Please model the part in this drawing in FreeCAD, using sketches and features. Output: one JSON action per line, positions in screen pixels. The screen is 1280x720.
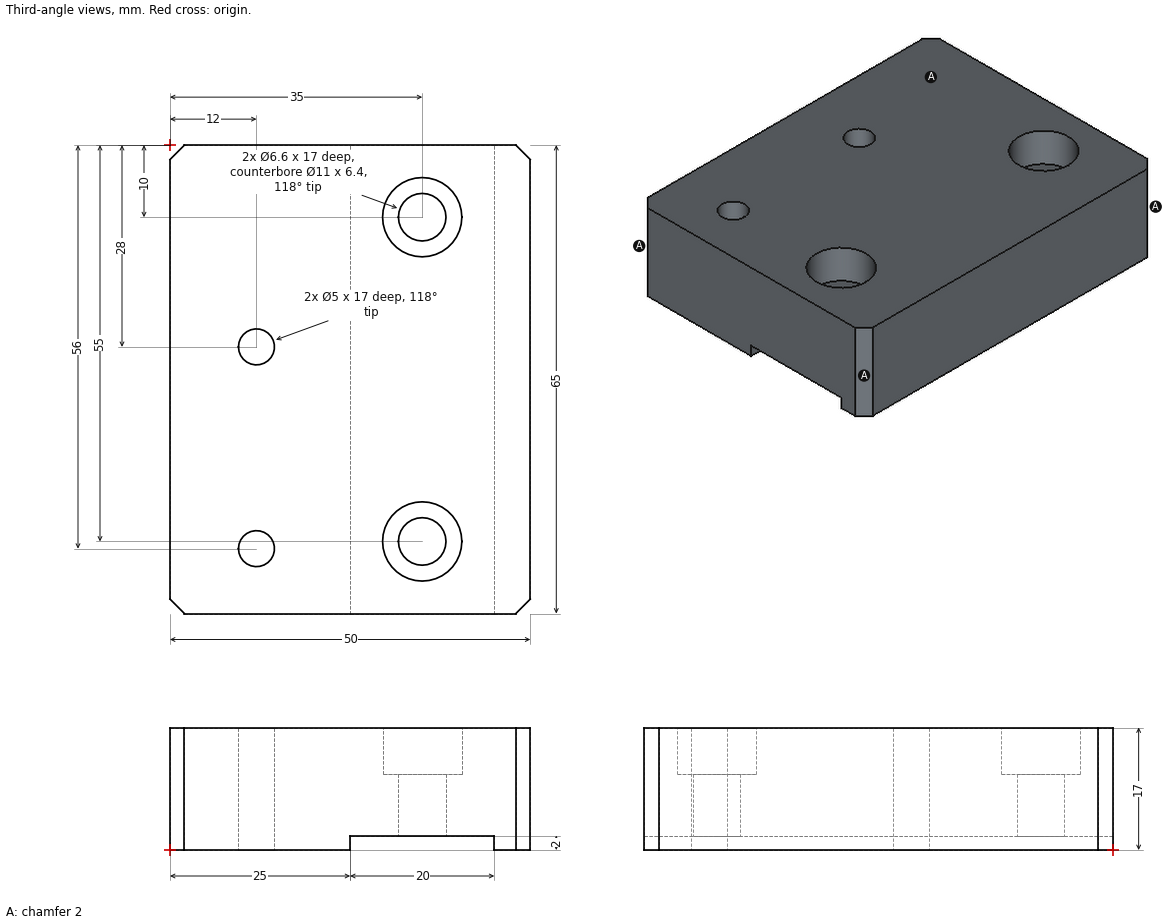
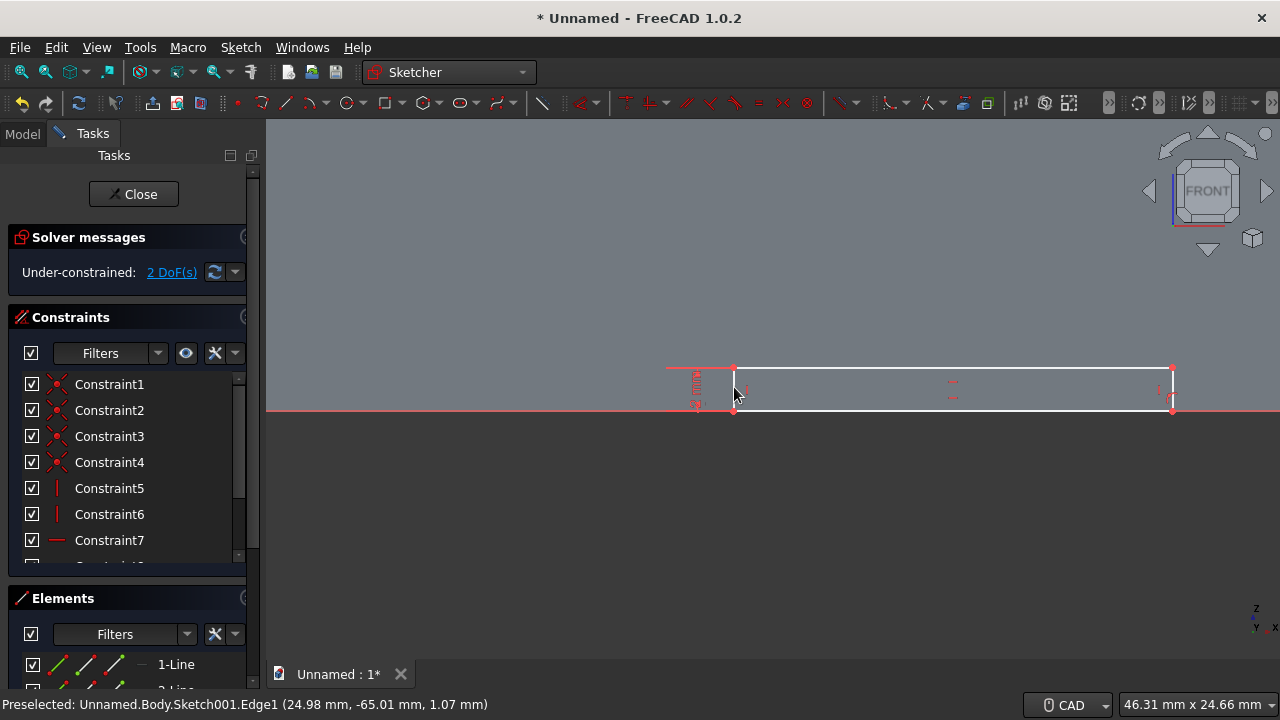
{"action": "left_click", "coordinate": [865, 411]}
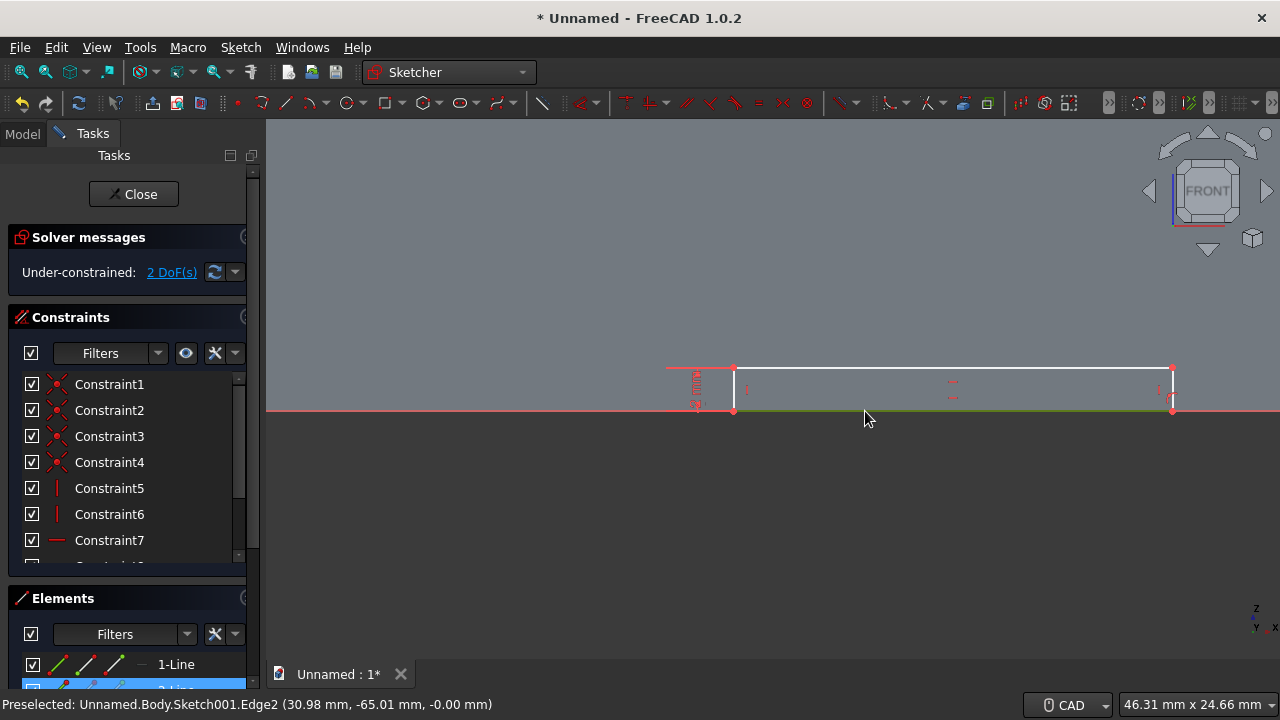
{"action": "key", "text": "l"}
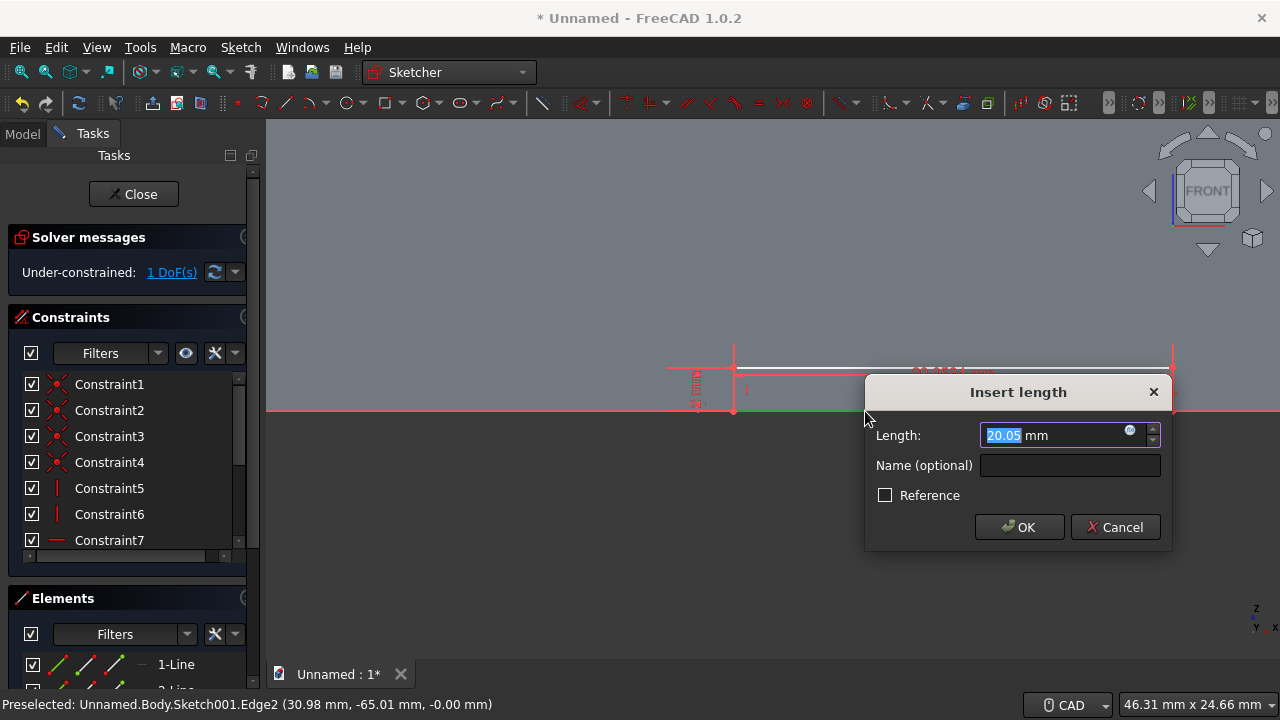
{"action": "type", "text": "20"}
{"action": "key", "text": "Return"}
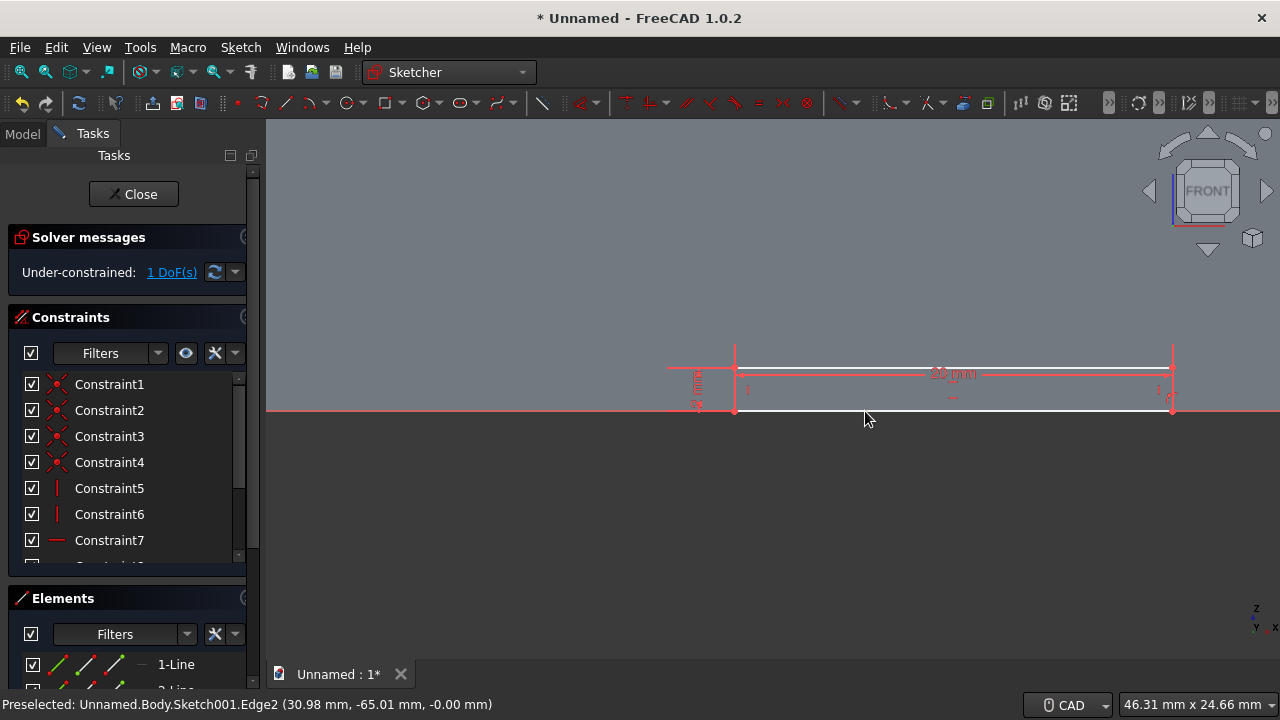
{"action": "left_click", "coordinate": [735, 368]}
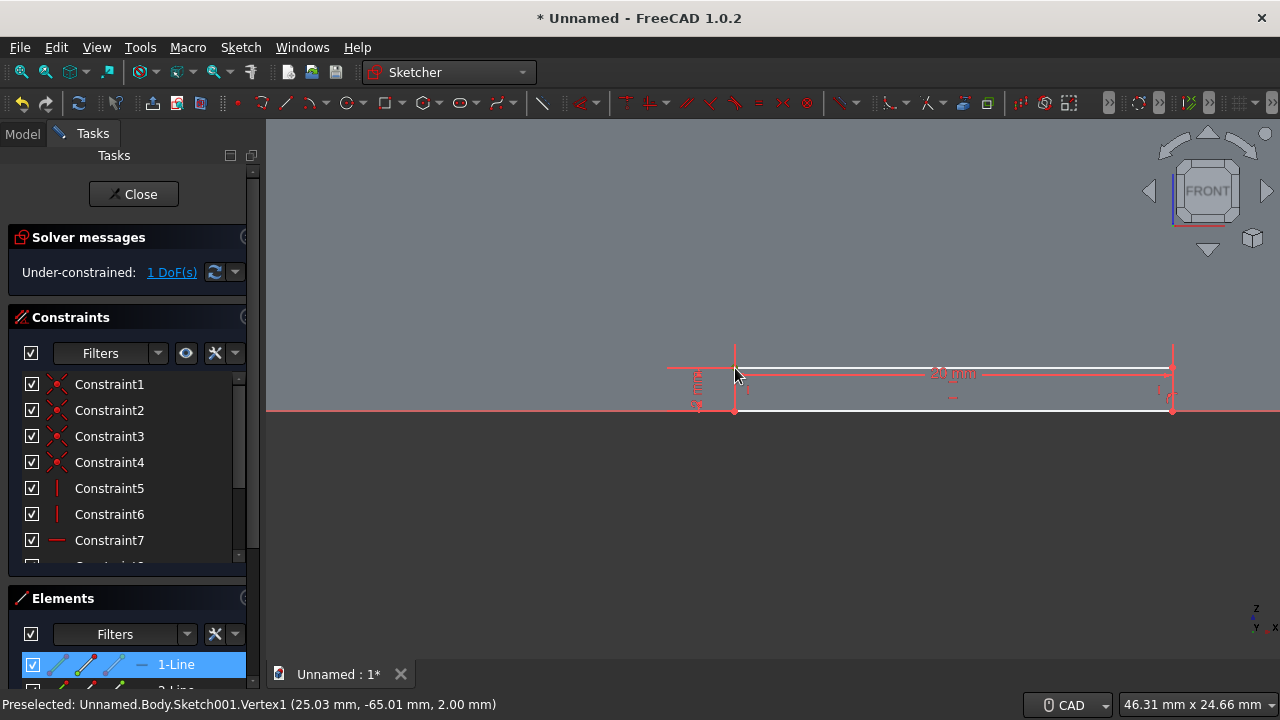
{"action": "left_click", "coordinate": [598, 104]}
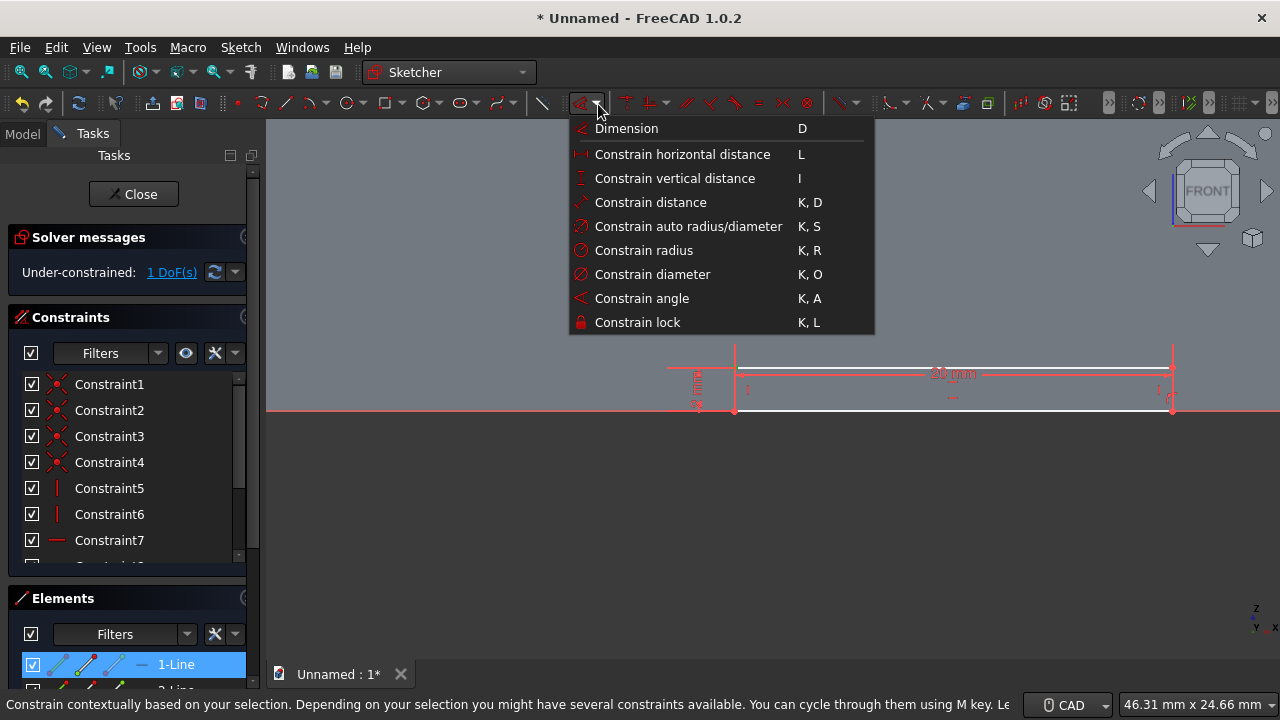
{"action": "left_click", "coordinate": [722, 154]}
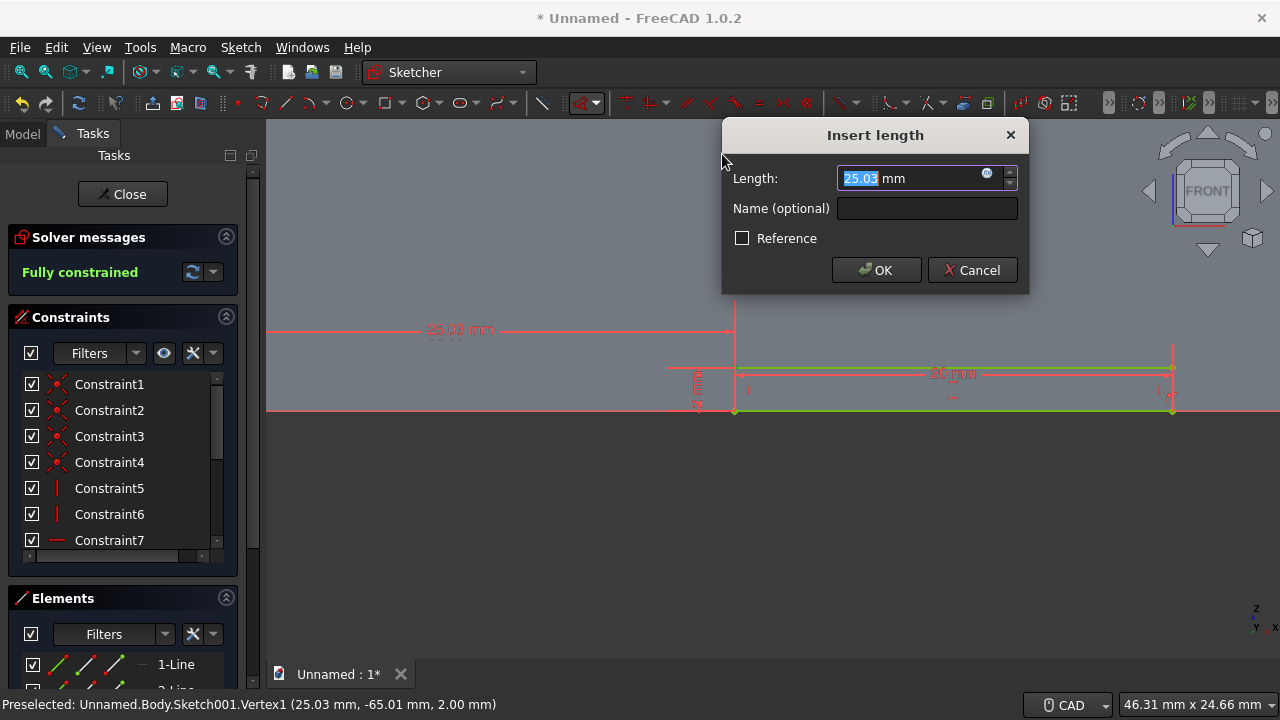
{"action": "type", "text": "25"}
{"action": "key", "text": "Return"}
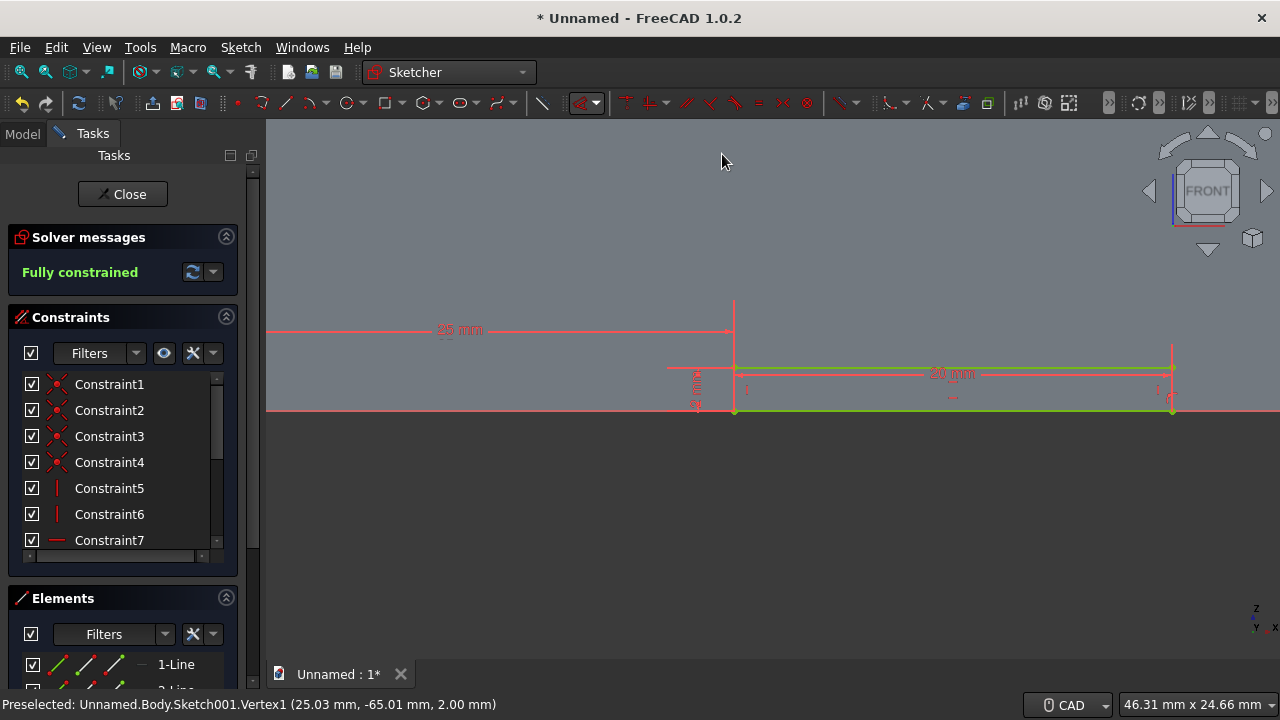
{"action": "left_click", "coordinate": [123, 194]}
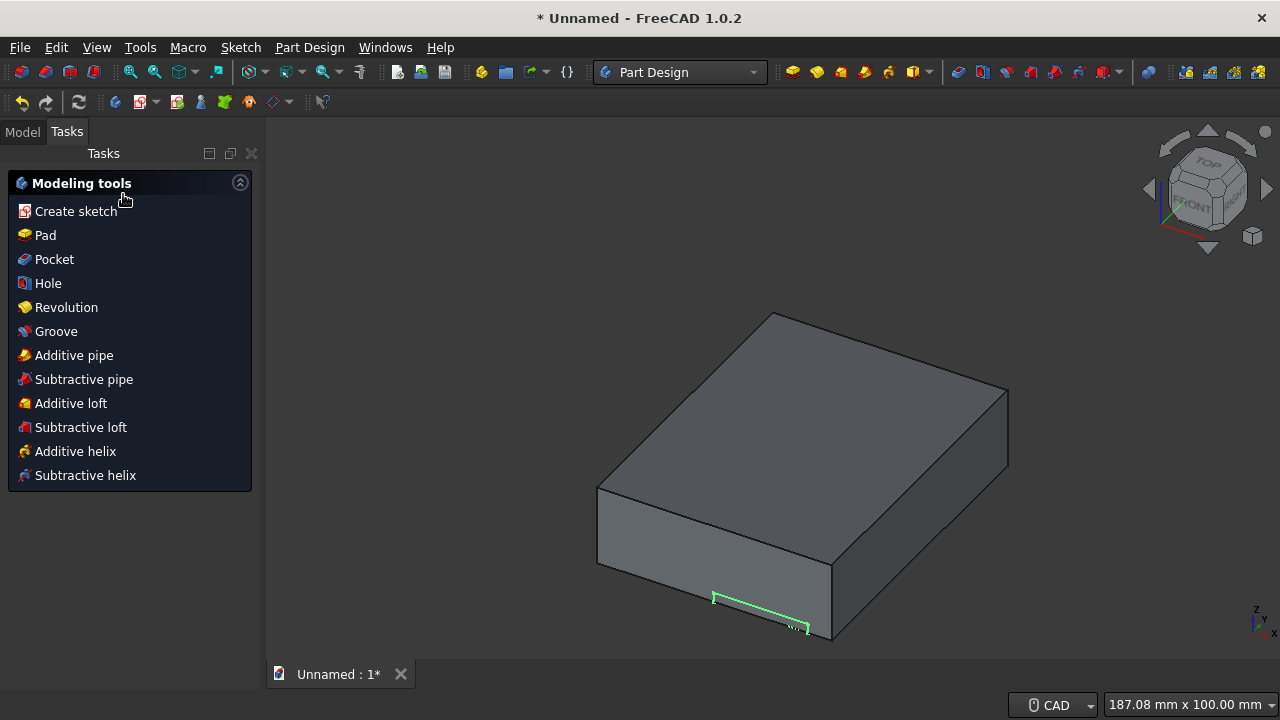
{"action": "left_click", "coordinate": [960, 72]}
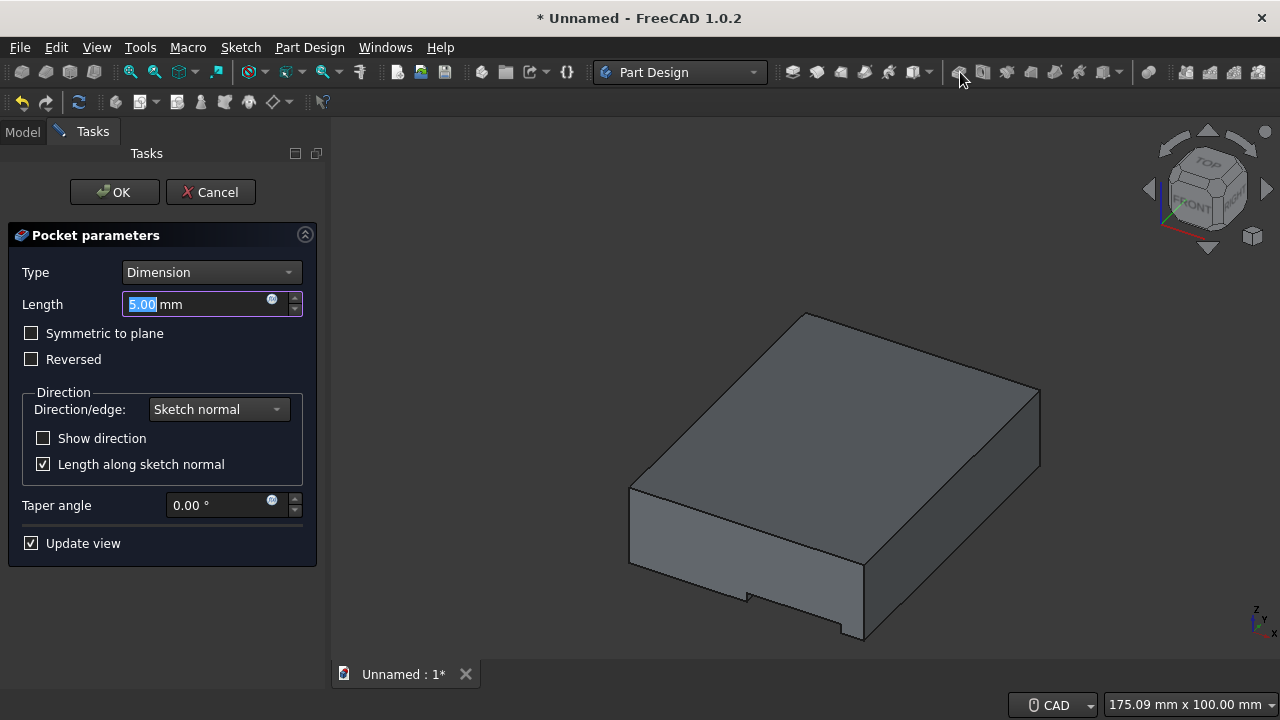
{"action": "left_click", "coordinate": [212, 272]}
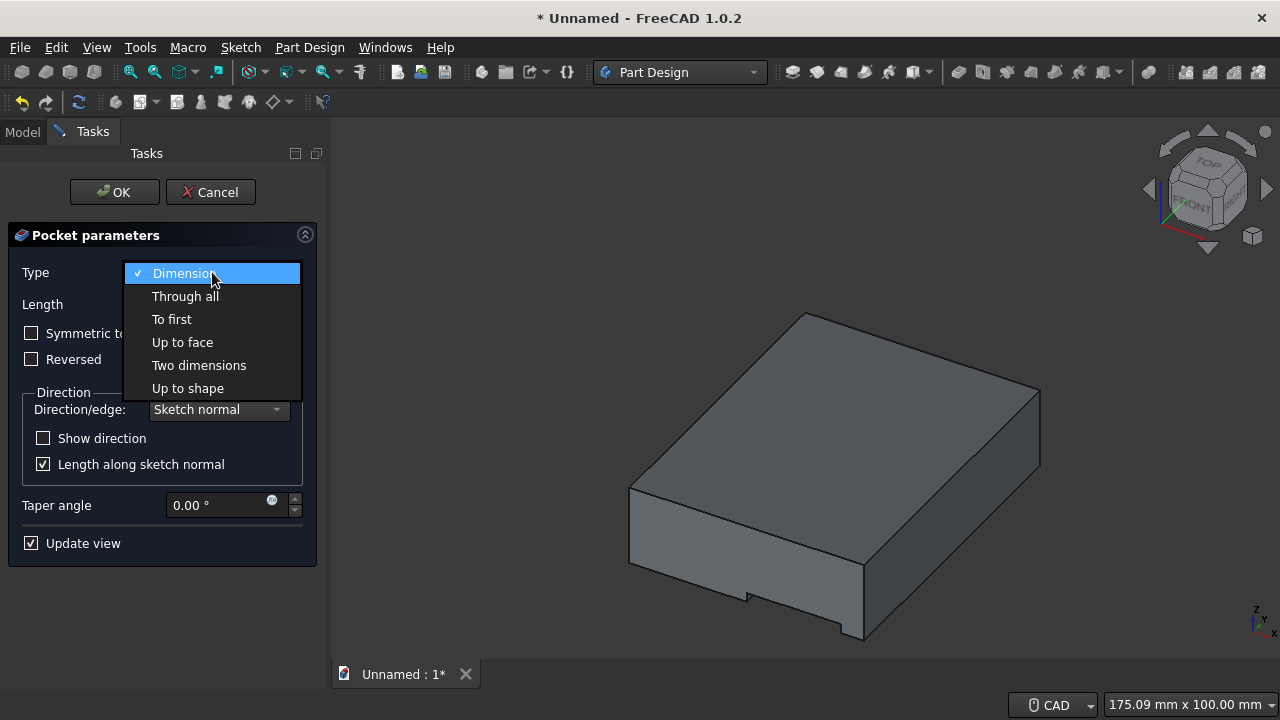
{"action": "left_click", "coordinate": [212, 296]}